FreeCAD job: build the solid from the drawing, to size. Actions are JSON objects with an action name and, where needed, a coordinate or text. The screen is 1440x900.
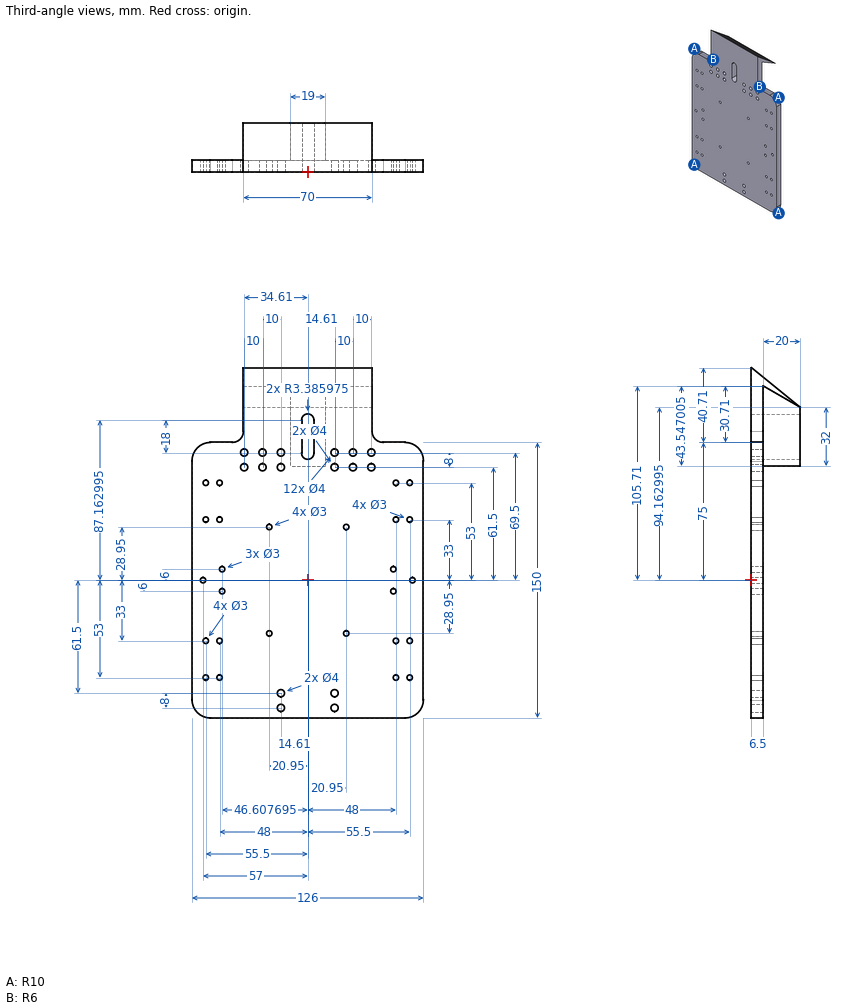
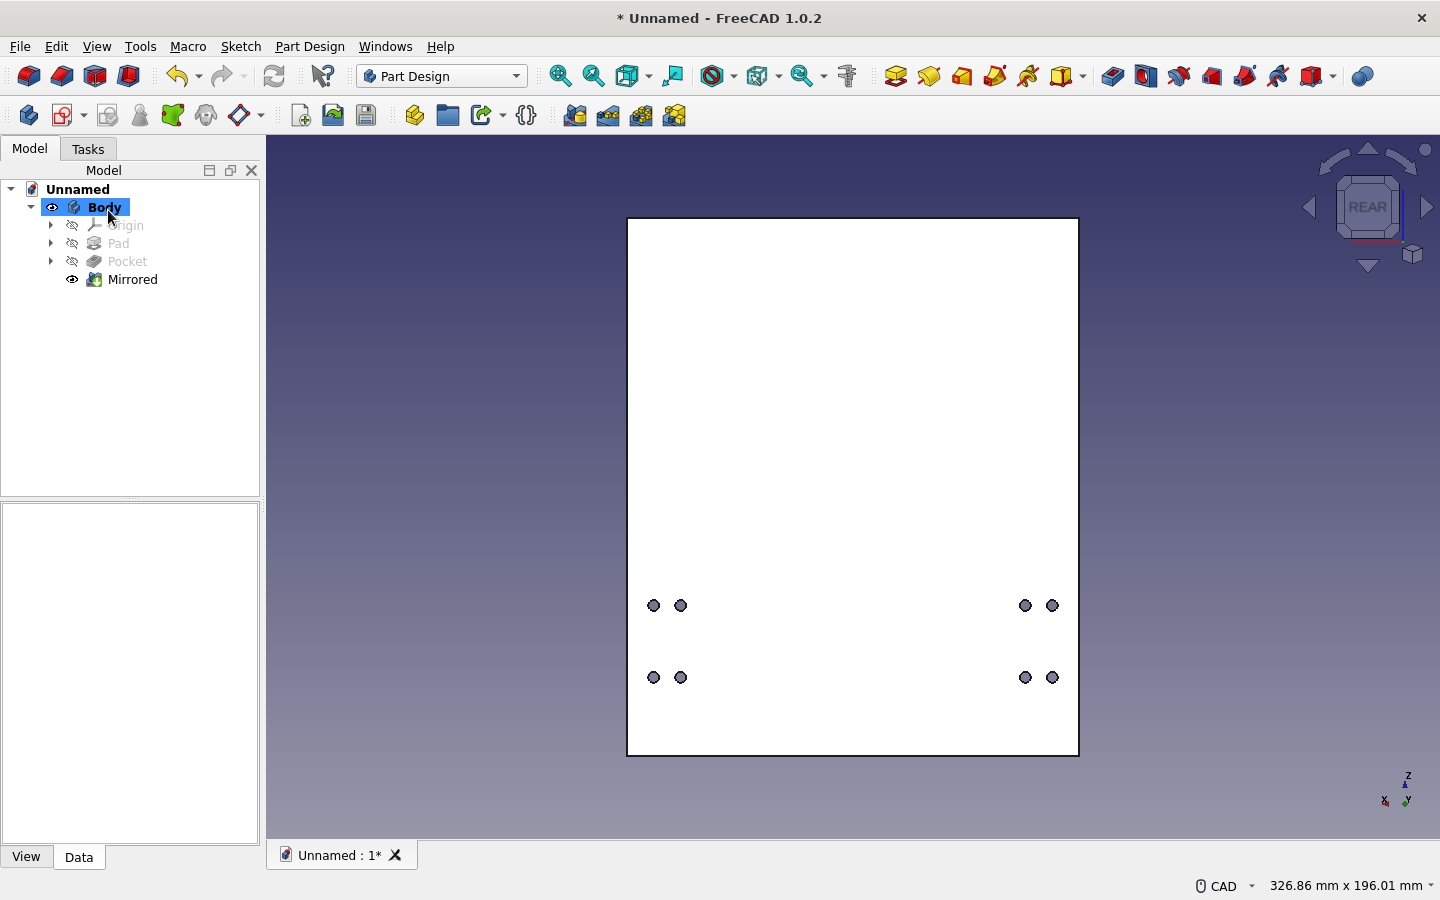
{"action": "left_click", "coordinate": [117, 261]}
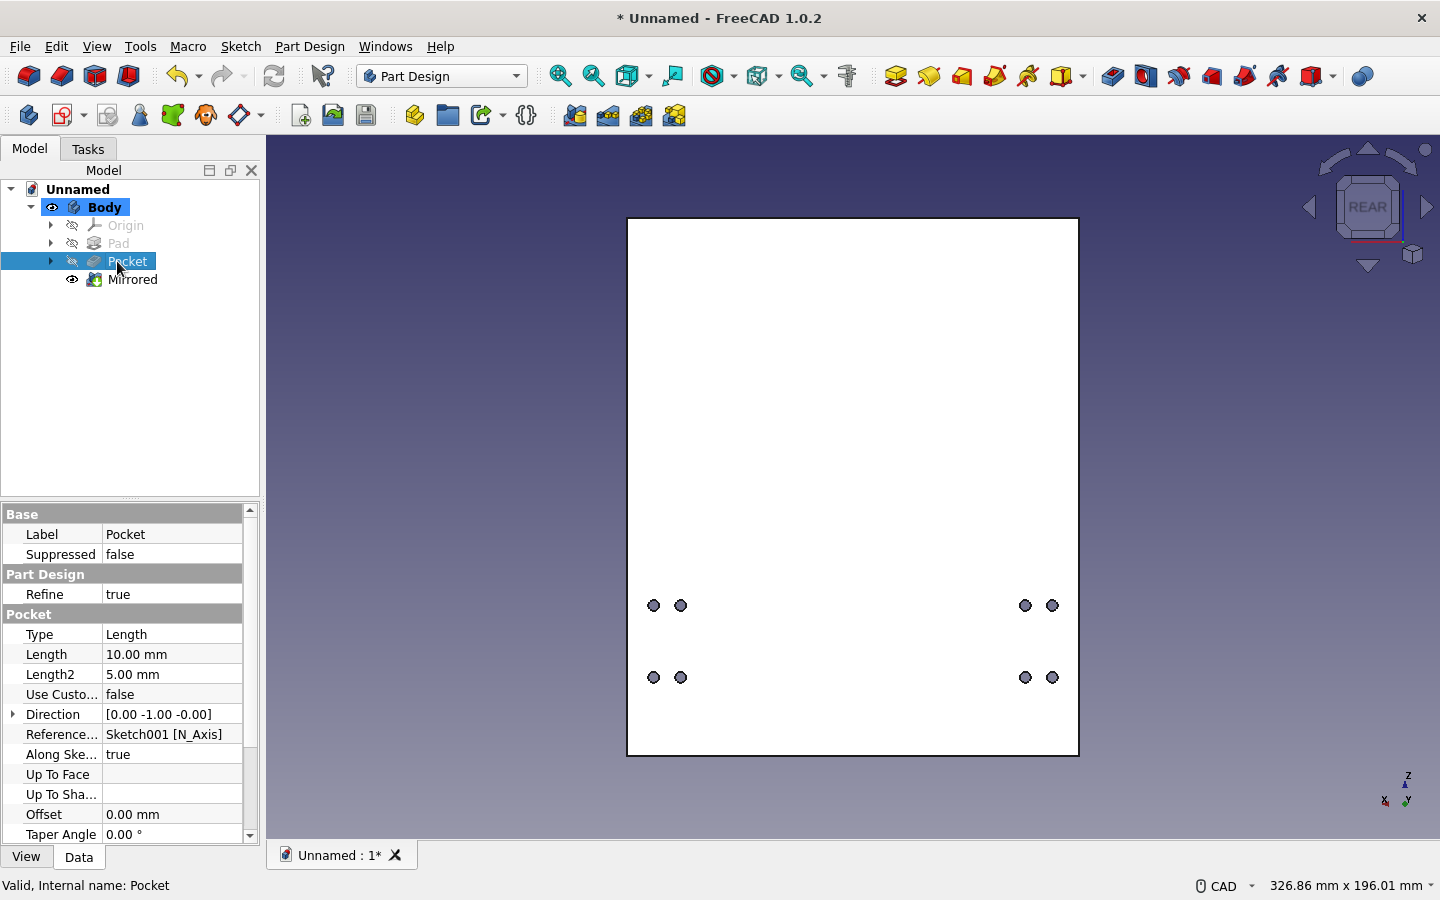
{"action": "left_click", "coordinate": [575, 116]}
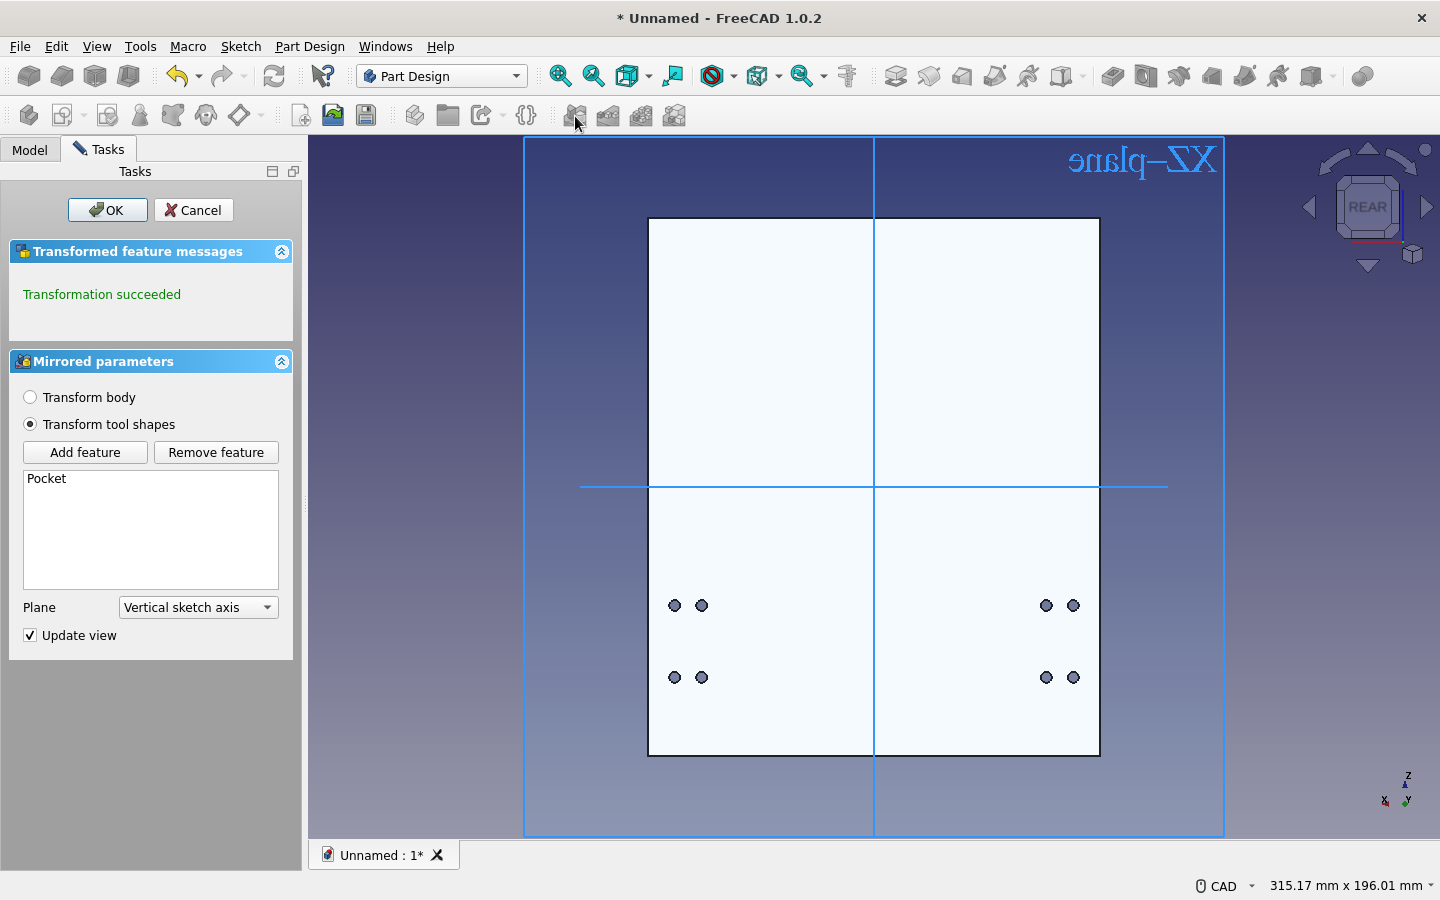
{"action": "left_click", "coordinate": [199, 608]}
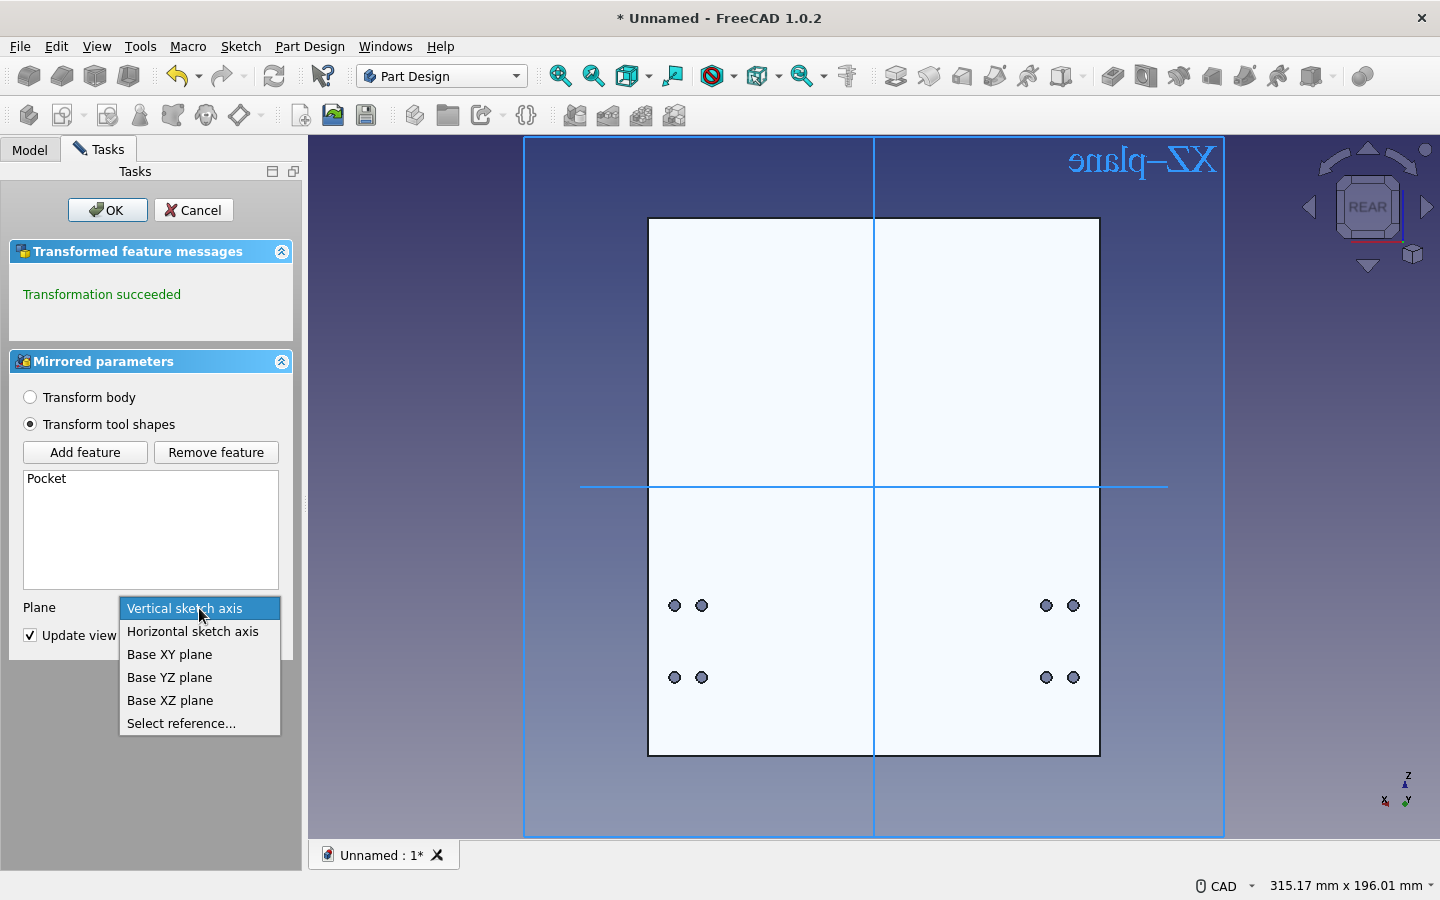
{"action": "left_click", "coordinate": [198, 654]}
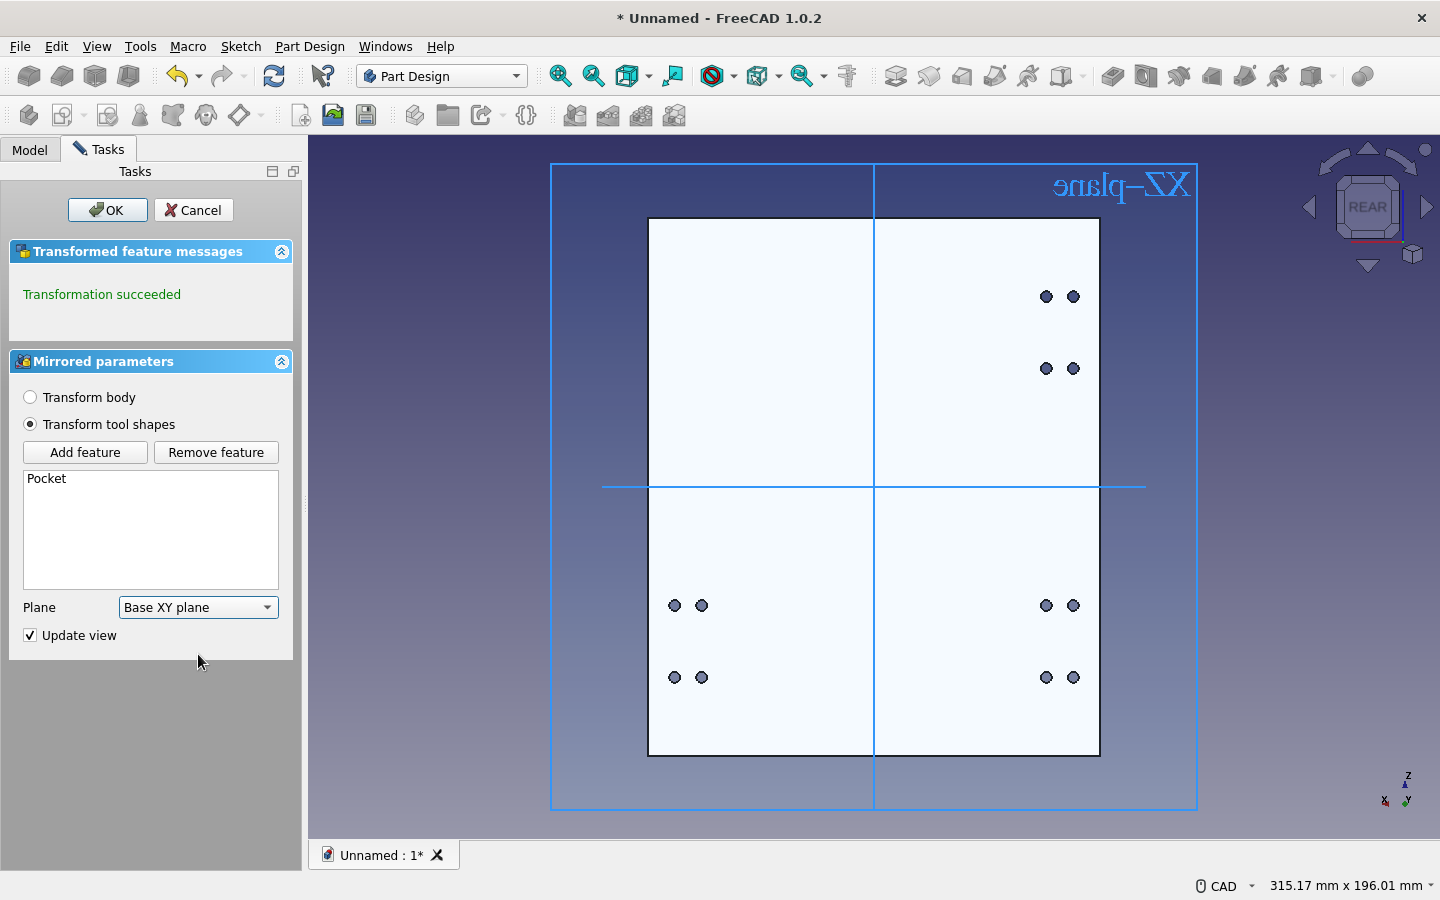
{"action": "left_click", "coordinate": [108, 210]}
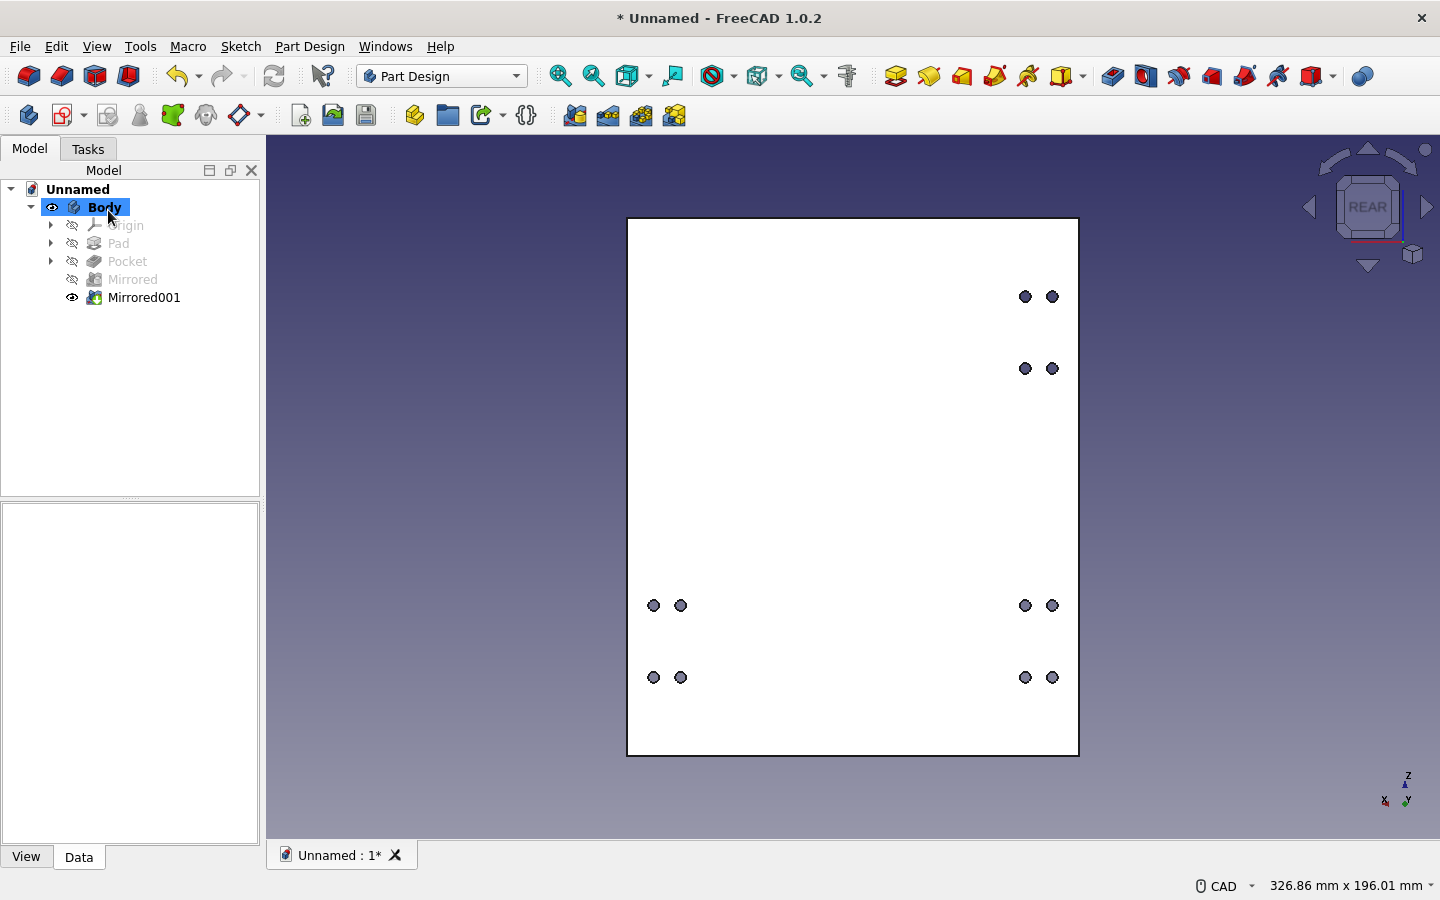
{"action": "left_click", "coordinate": [853, 486]}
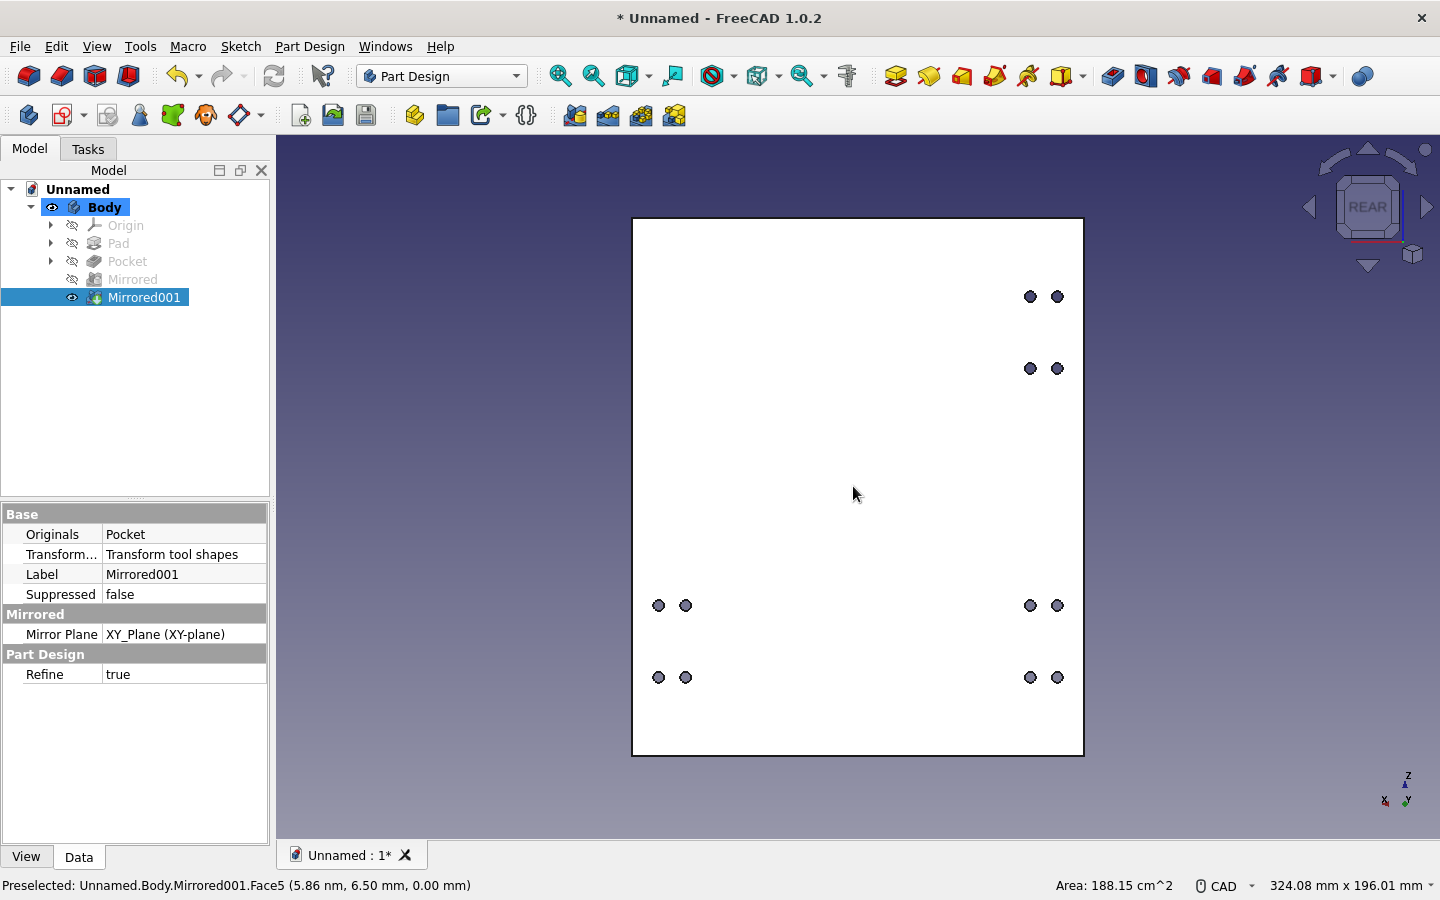
{"action": "left_click", "coordinate": [62, 116]}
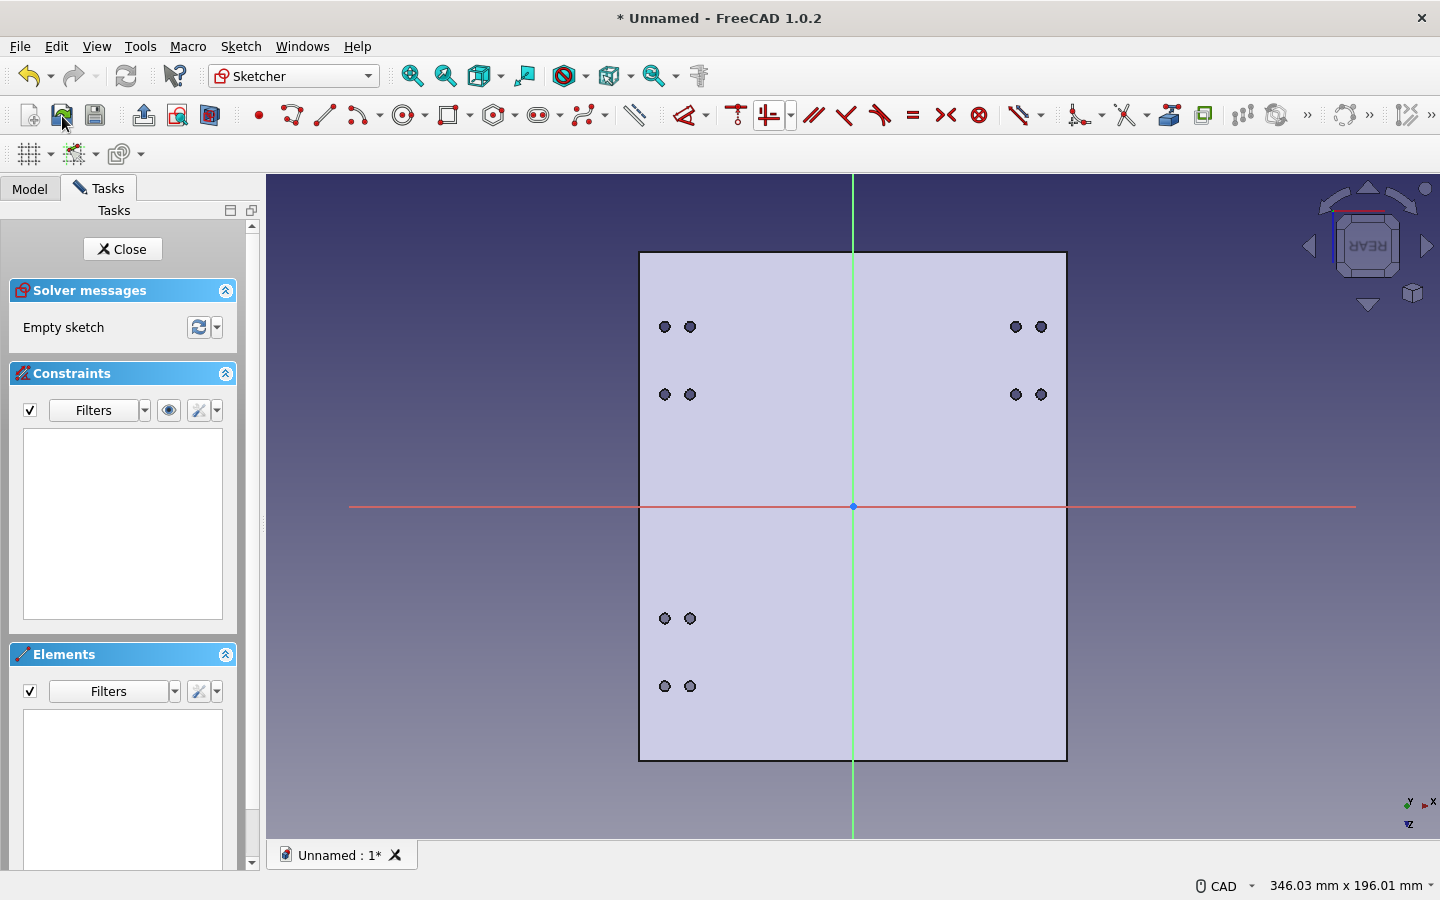
{"action": "scroll", "coordinate": [1084, 674], "scroll_direction": "up", "scroll_amount": 4}